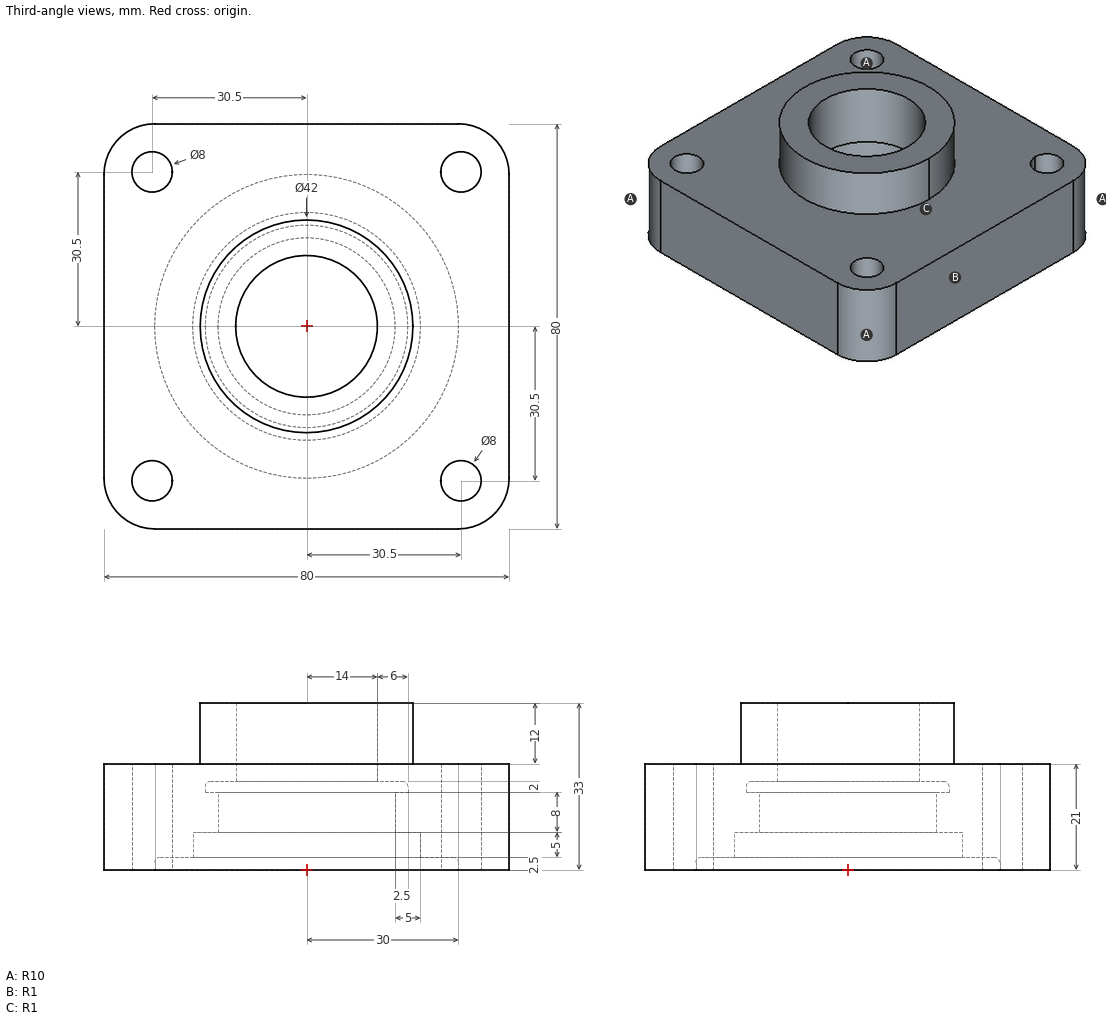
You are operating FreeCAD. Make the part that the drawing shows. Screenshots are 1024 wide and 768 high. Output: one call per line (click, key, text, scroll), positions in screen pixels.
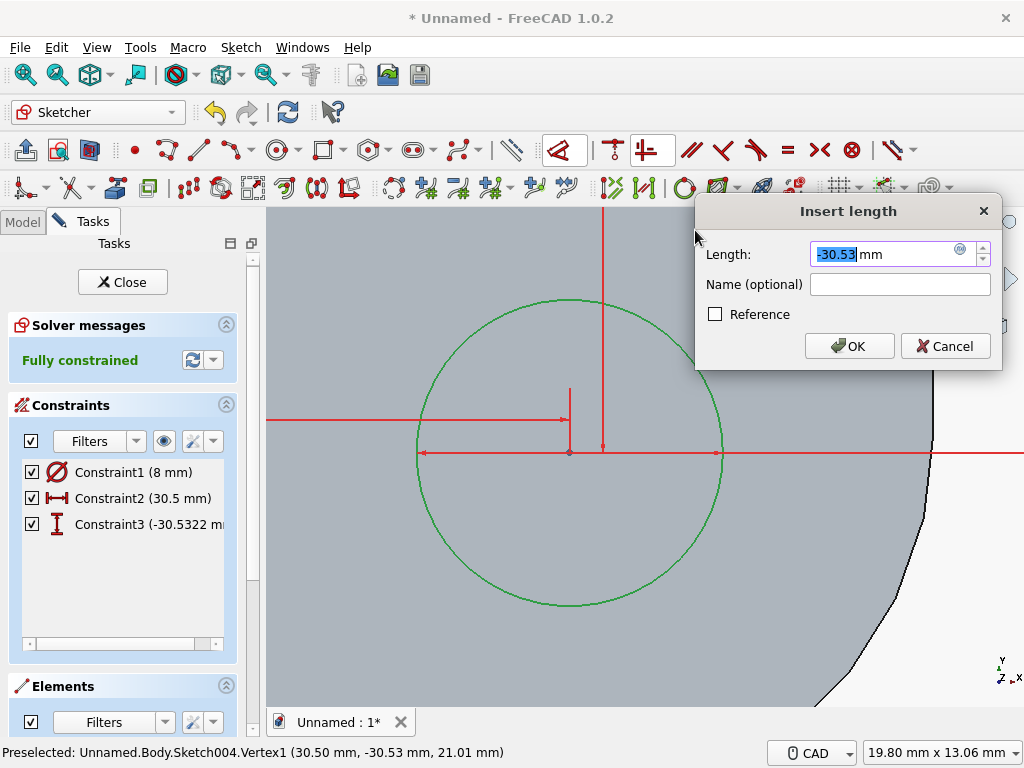
text(-30.5)
key(Return)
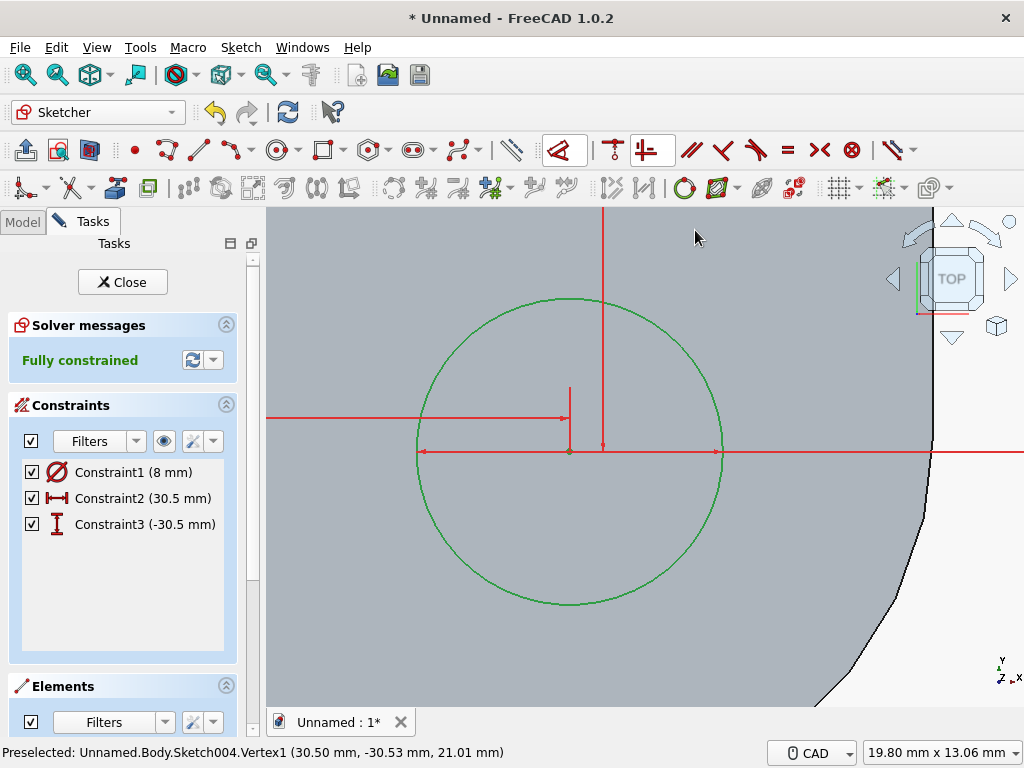
click(123, 282)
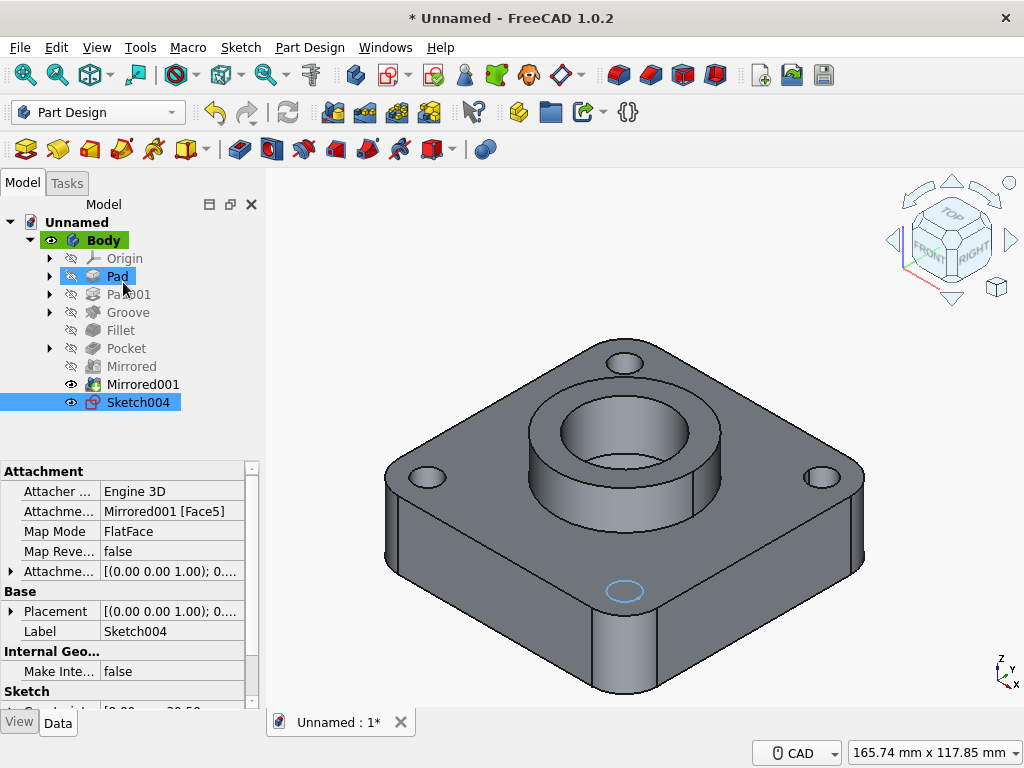
click(240, 150)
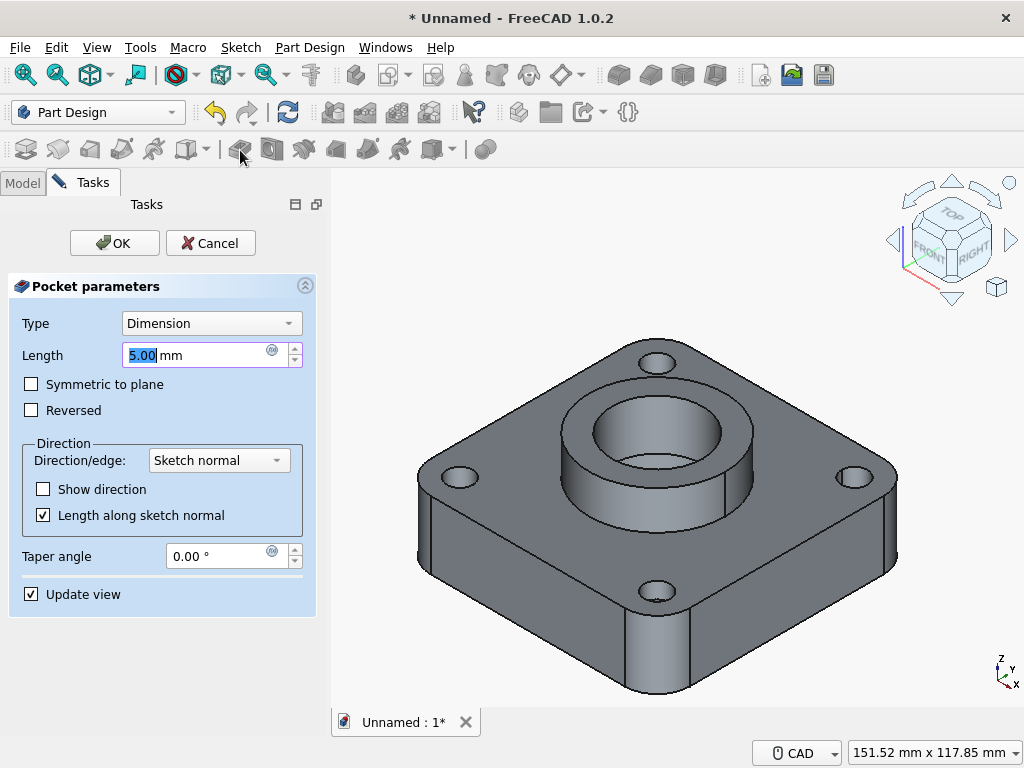
text(21)
key(Tab)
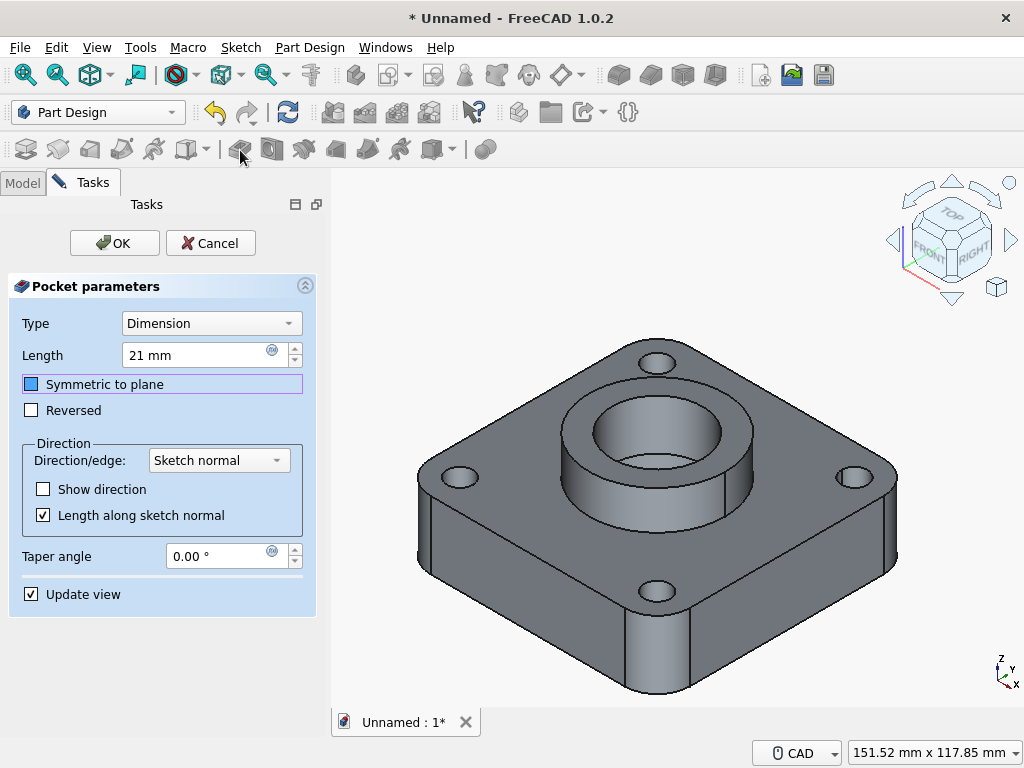
click(115, 243)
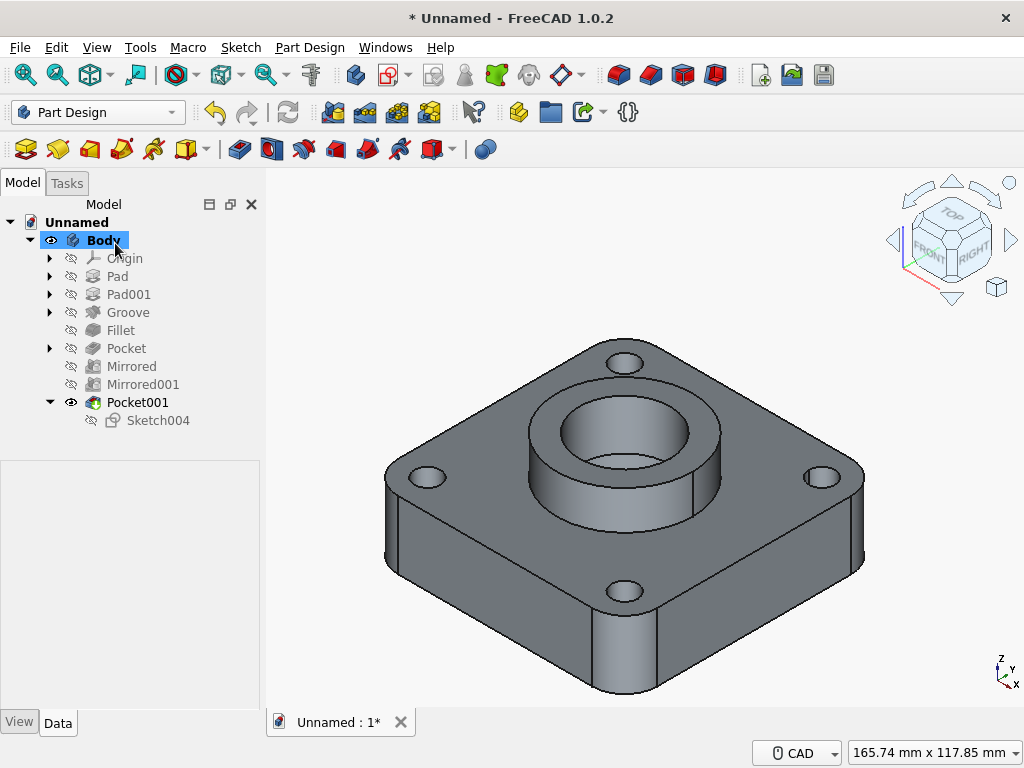
key(2)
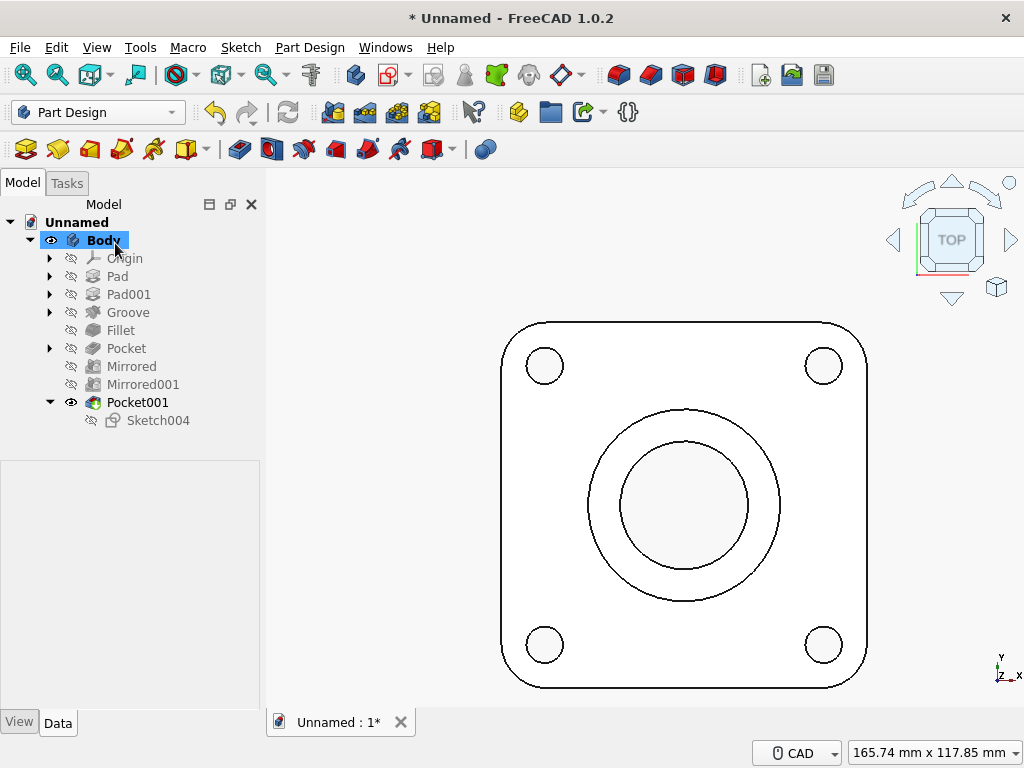
key(0)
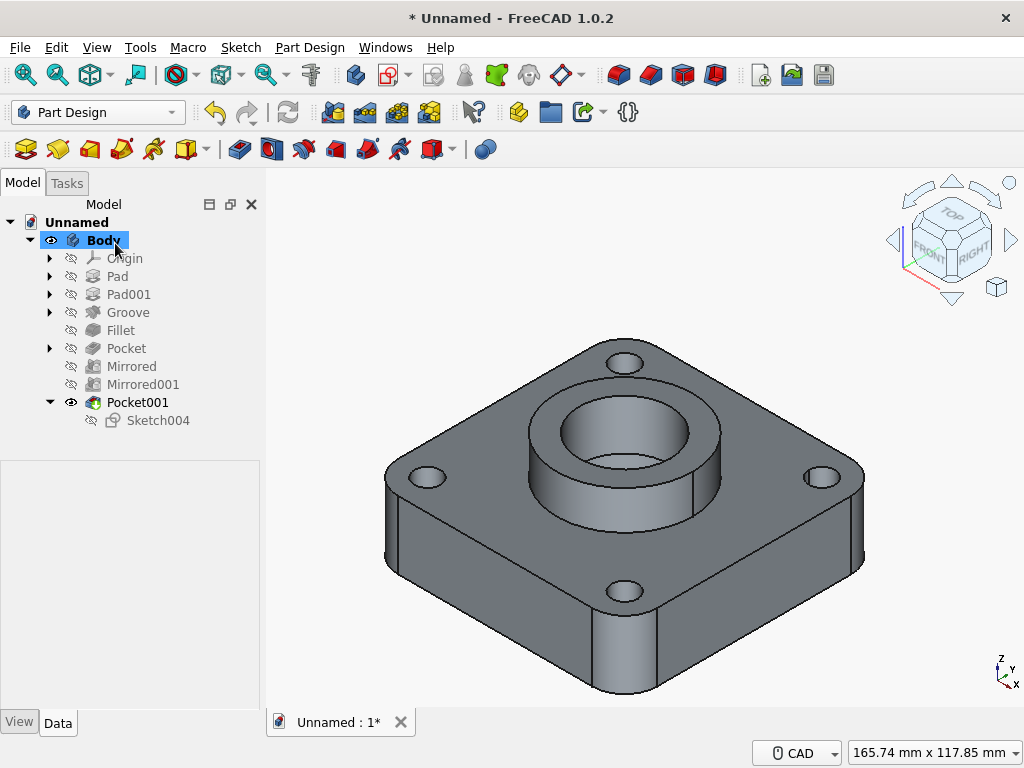
key(1)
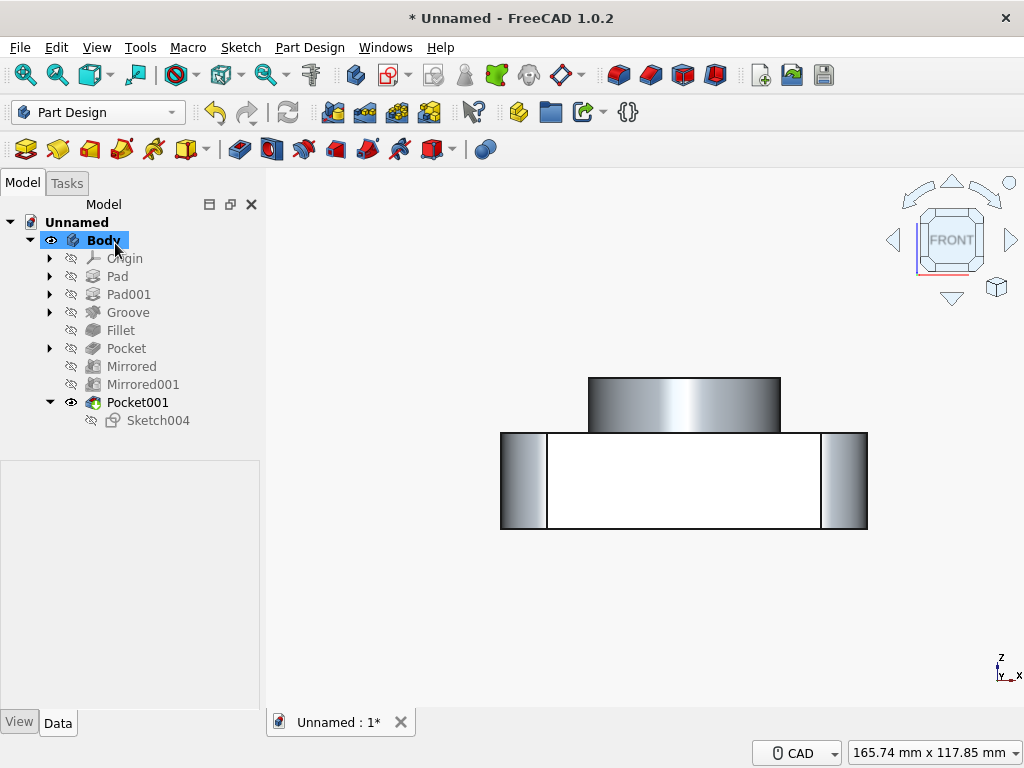
key(3)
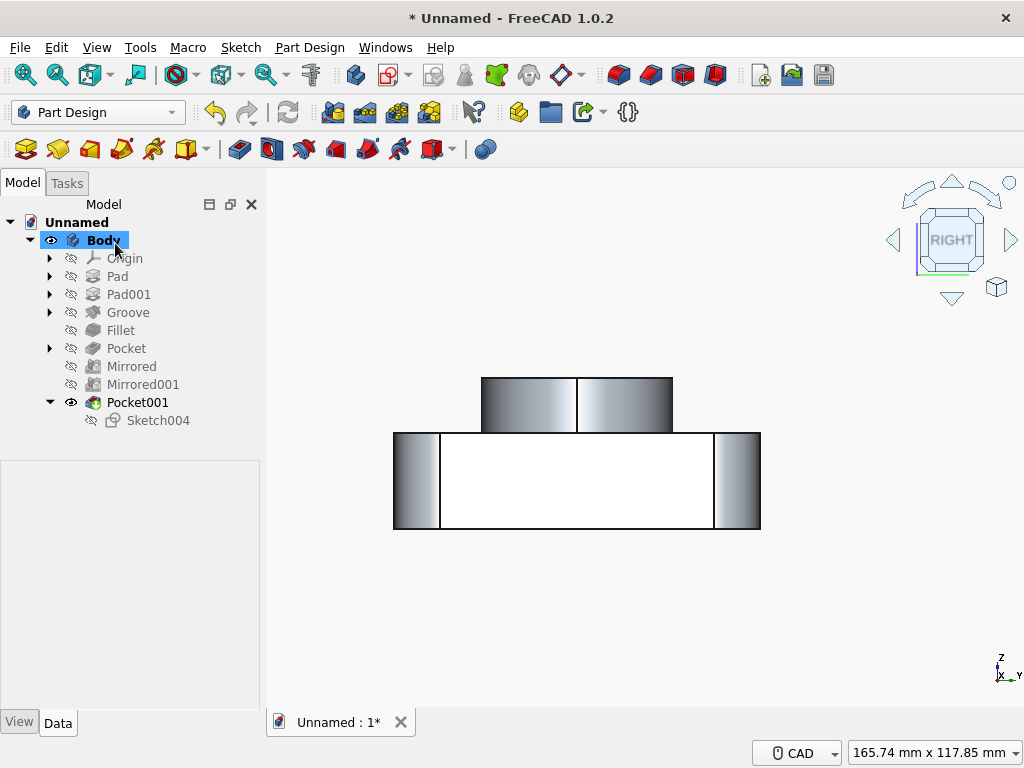
key(5)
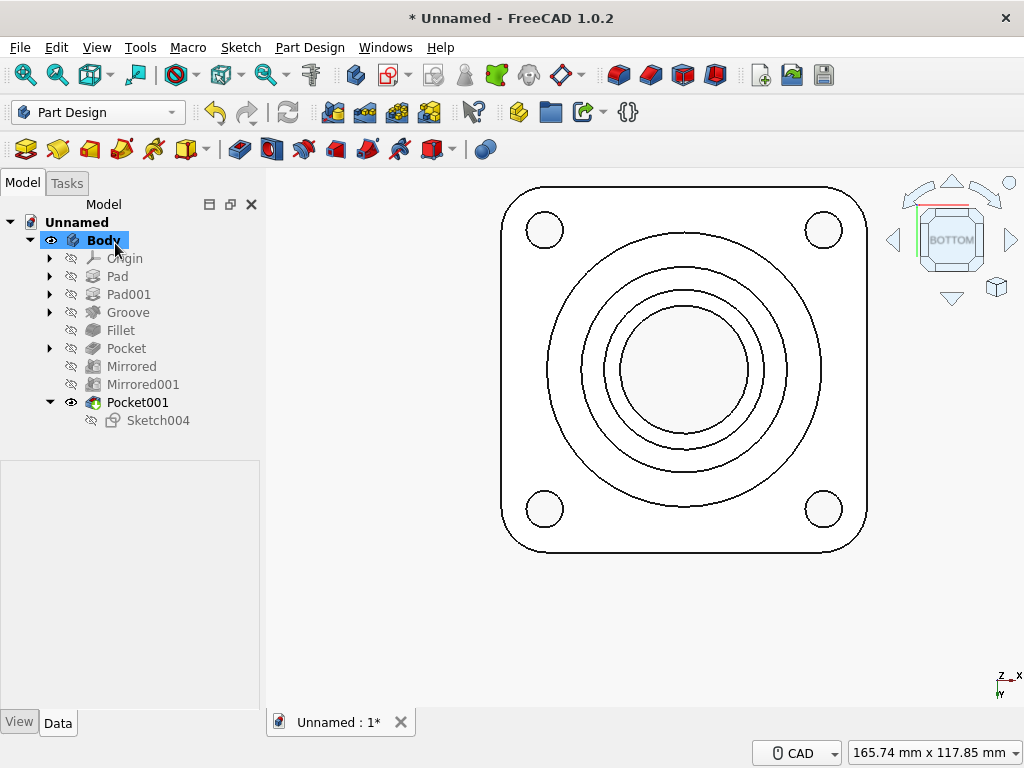
key(4)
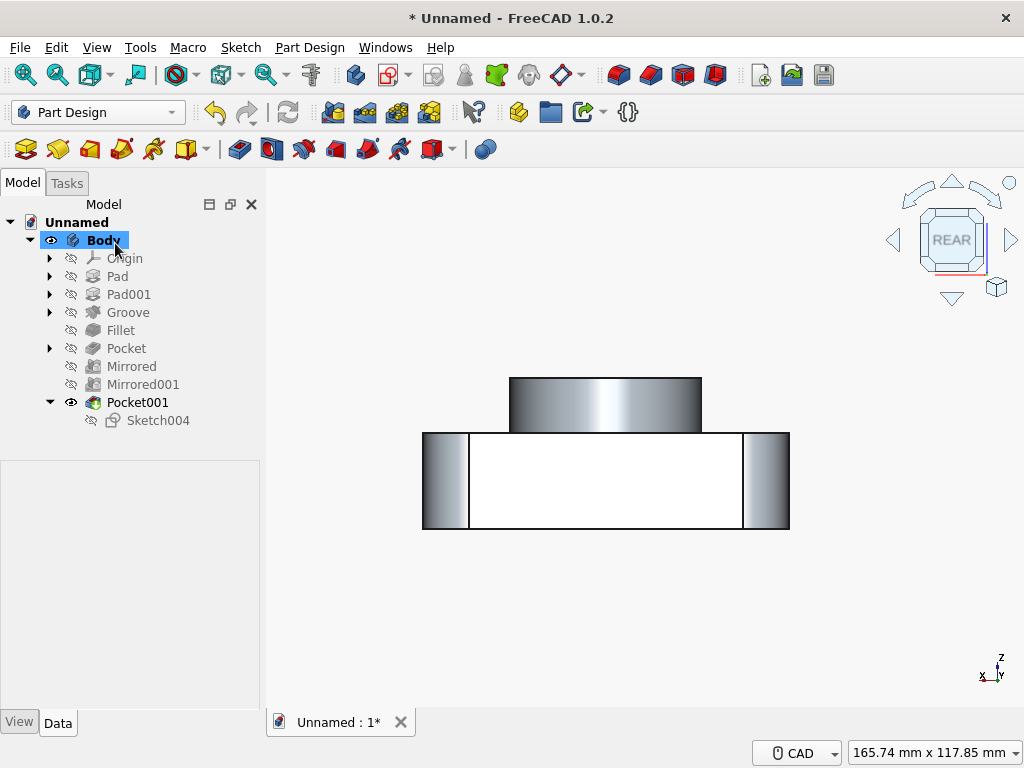
key(6)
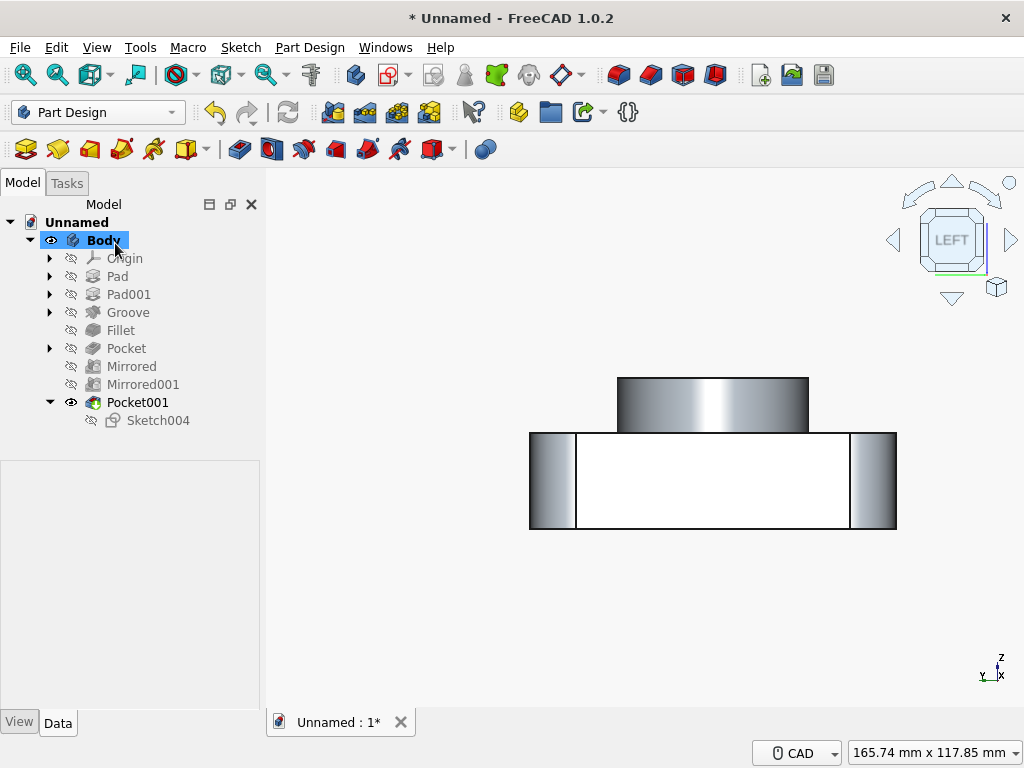
key(v)
key(3)